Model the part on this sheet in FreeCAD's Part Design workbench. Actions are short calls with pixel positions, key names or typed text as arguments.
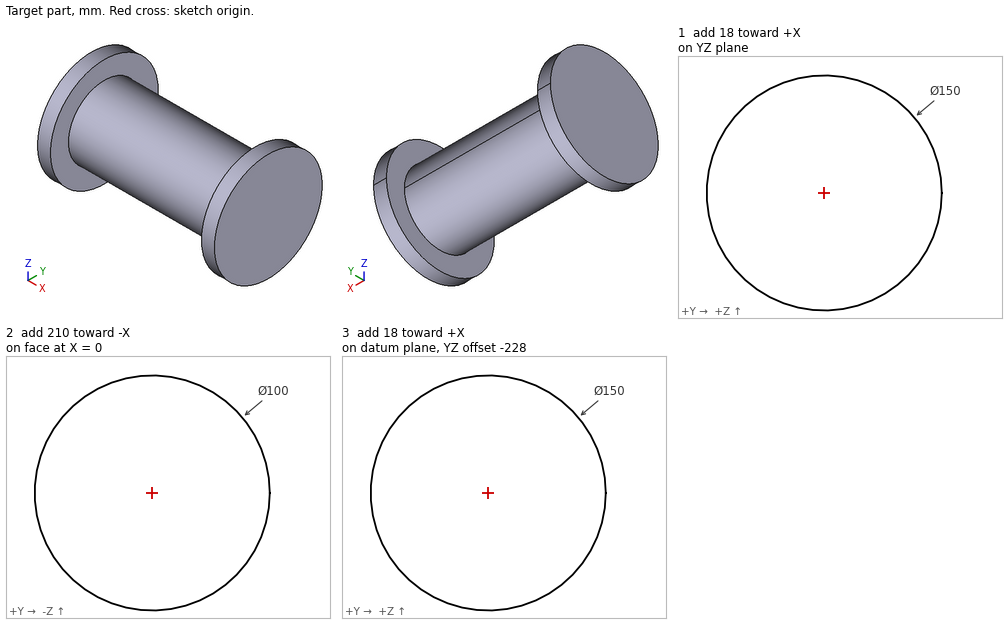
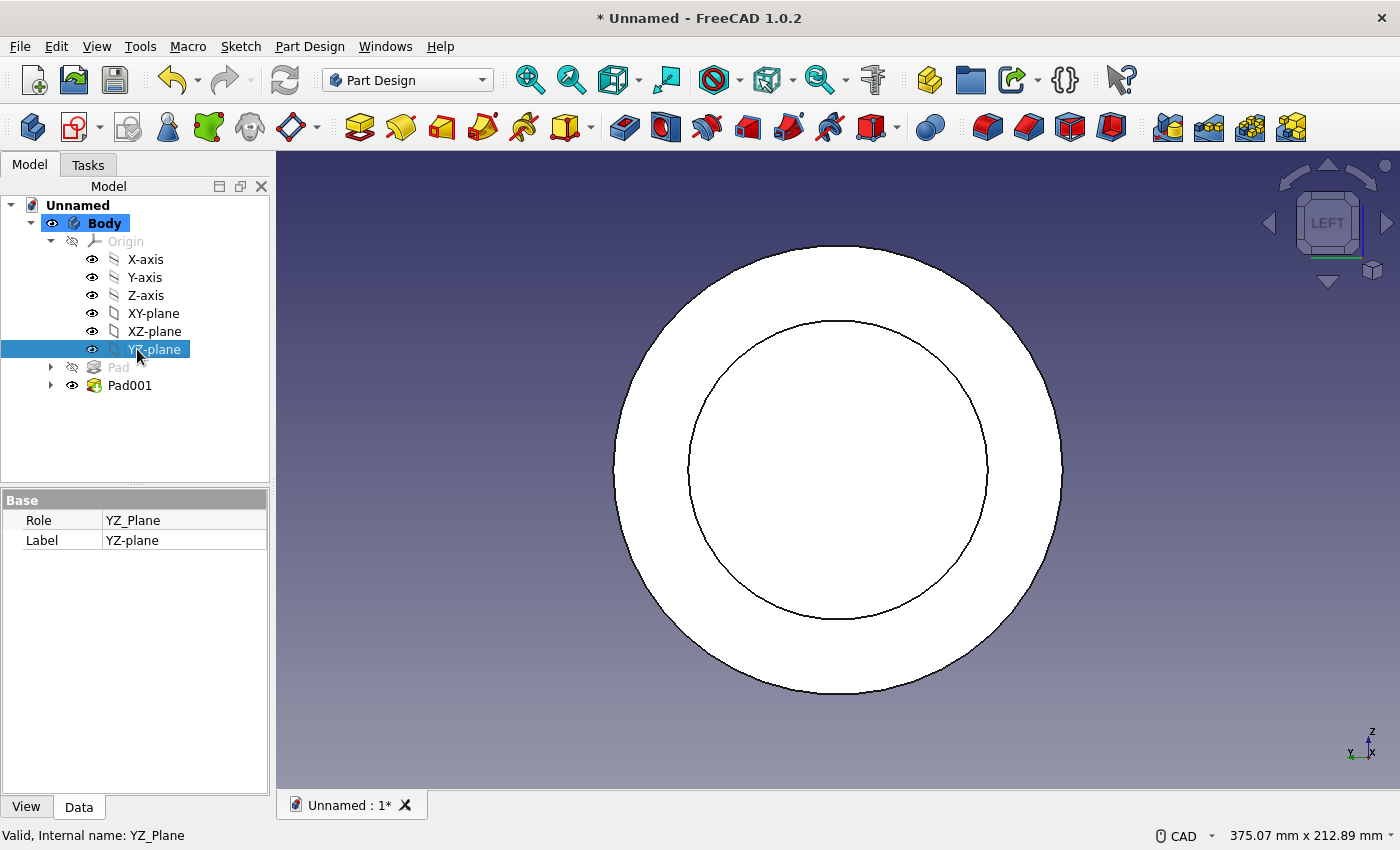
click(290, 128)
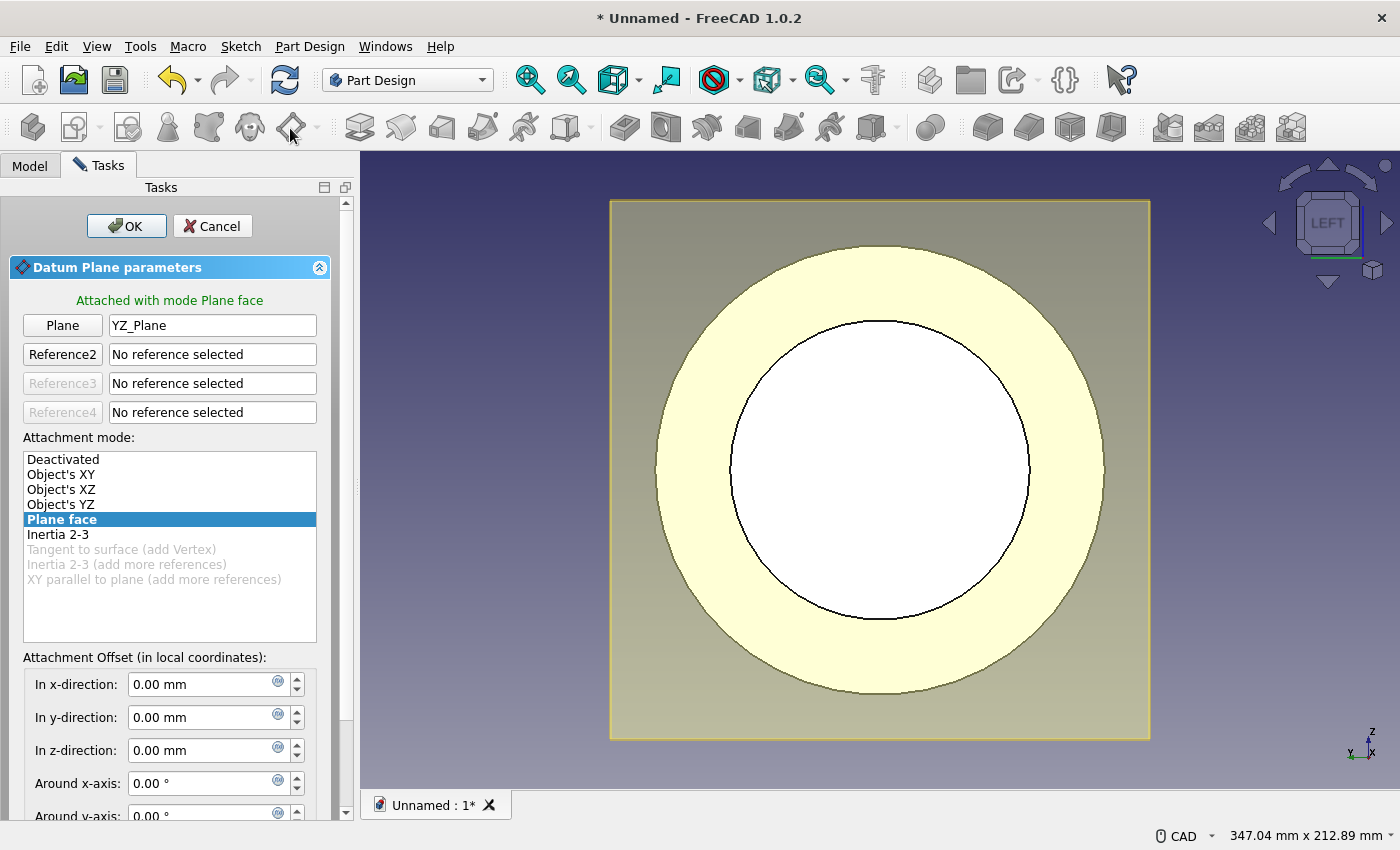
triple_click(210, 750)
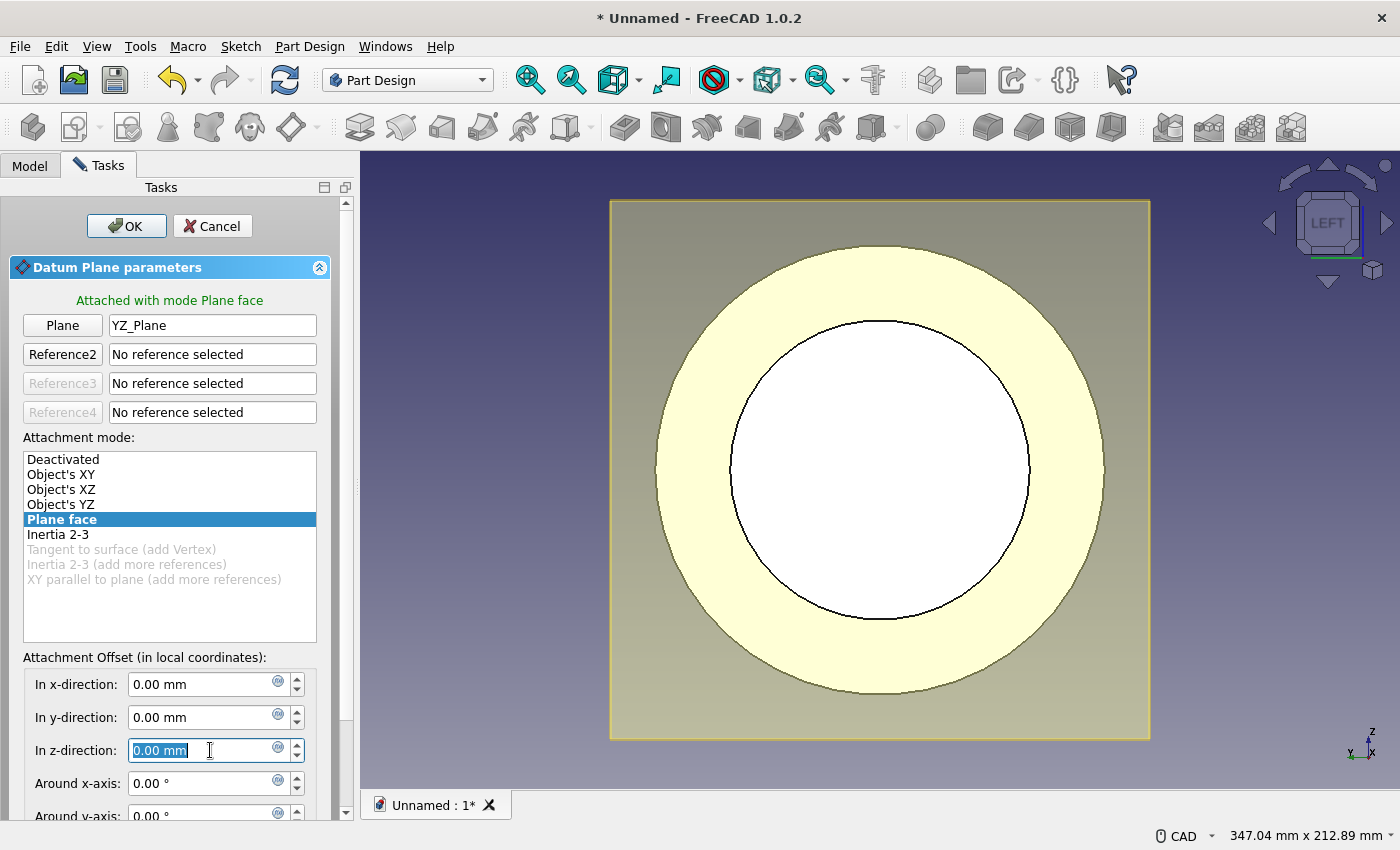
text(-228)
key(Tab)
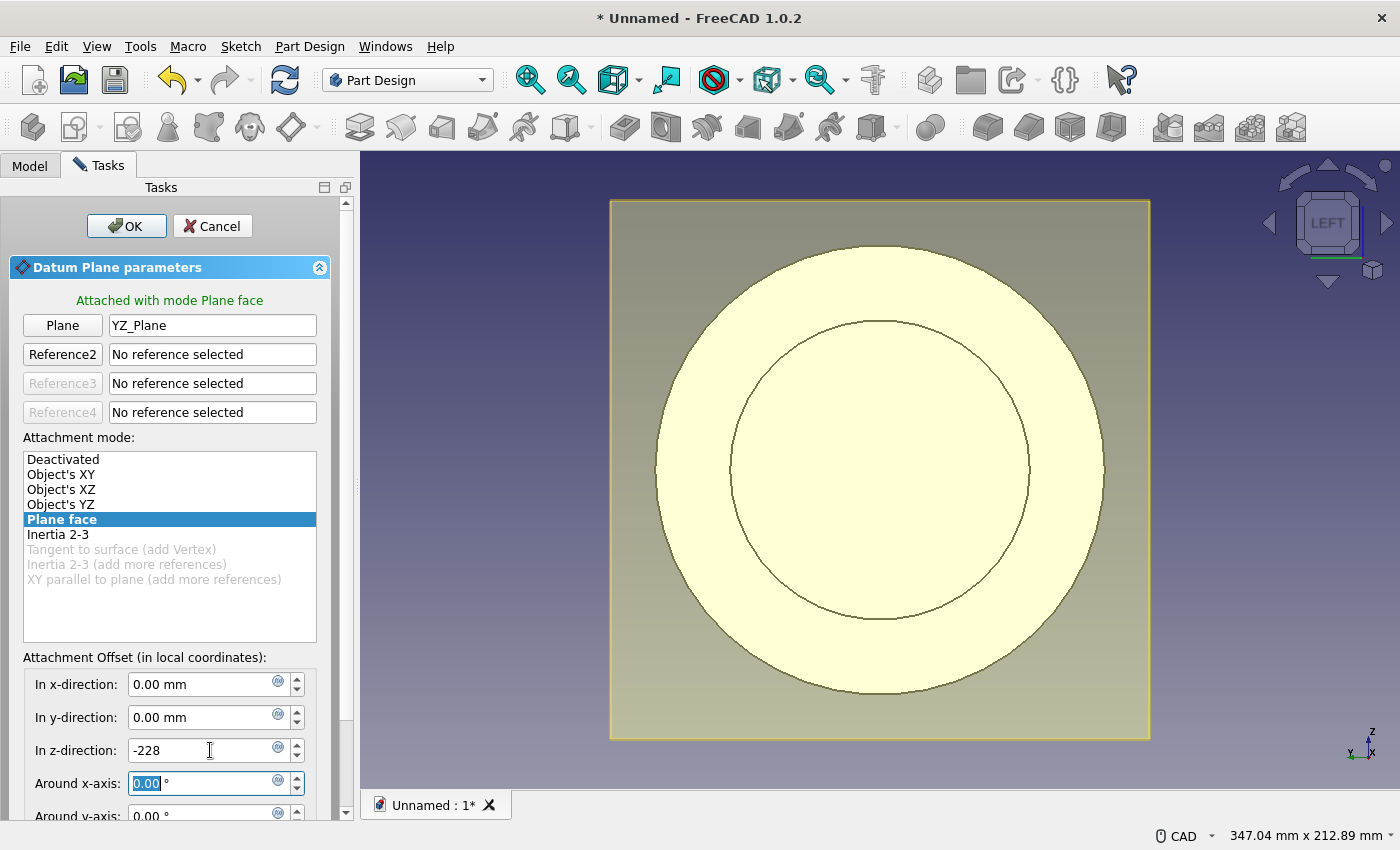
click(127, 226)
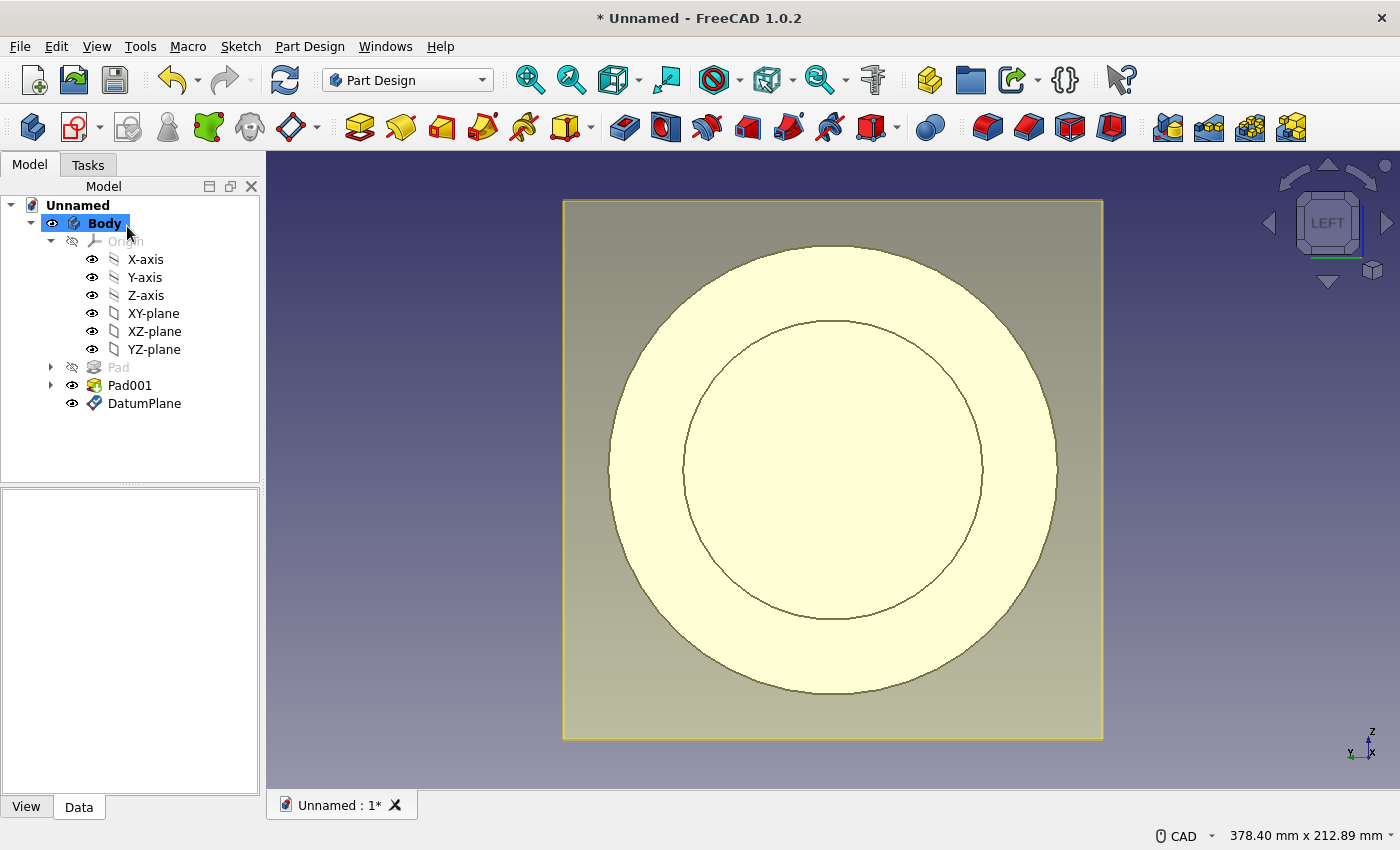
click(117, 403)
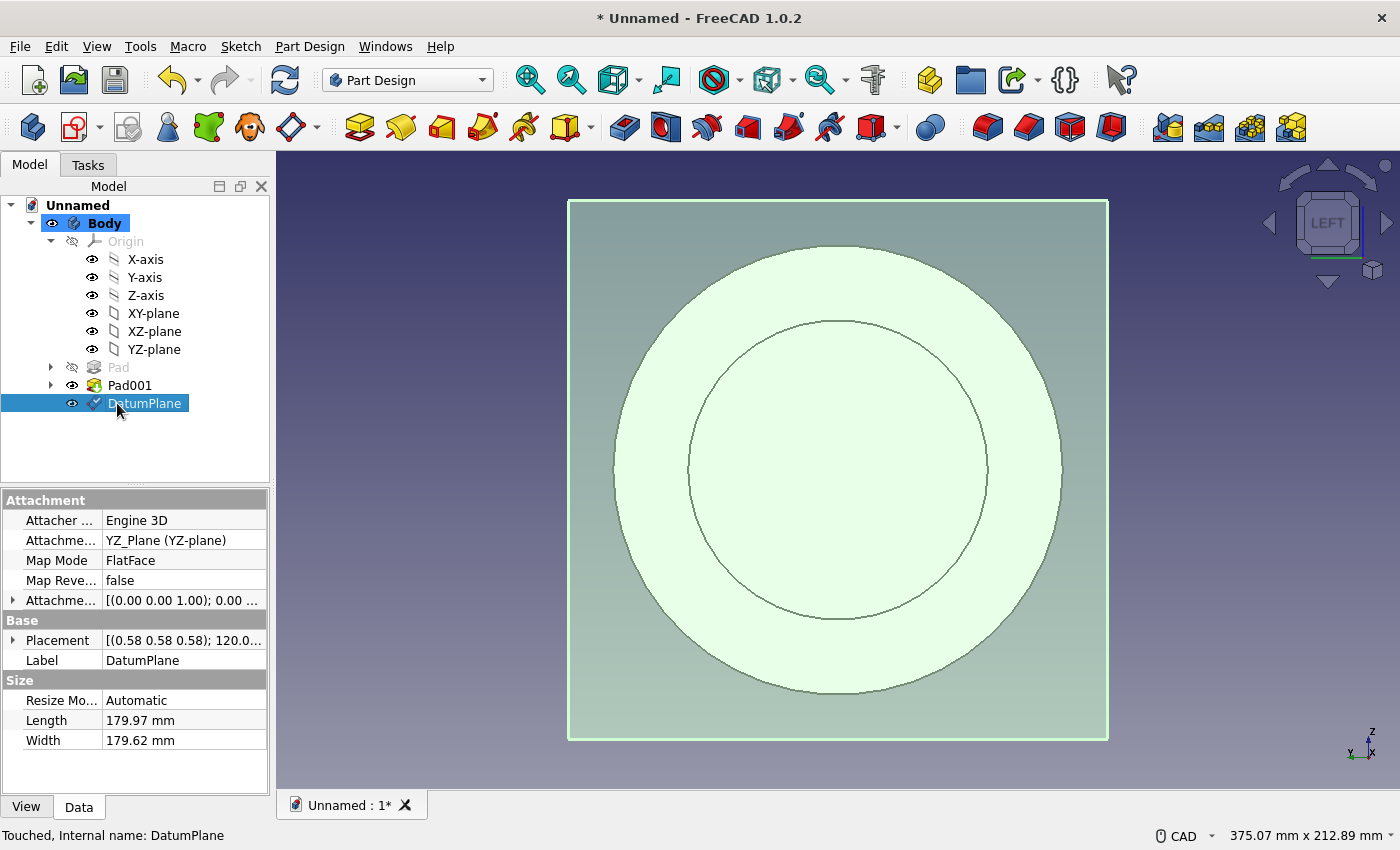
click(74, 128)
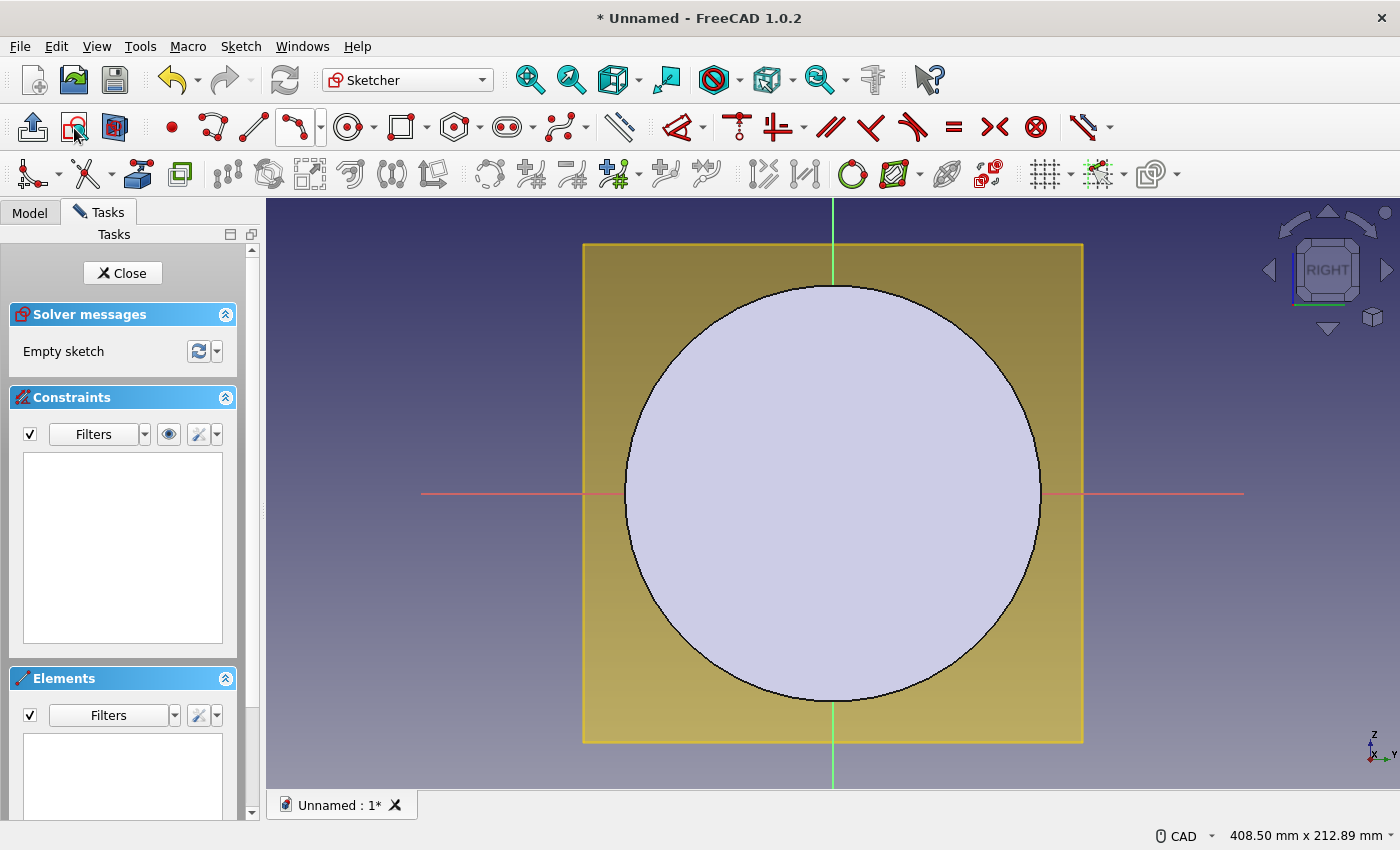
key(q)
key(s)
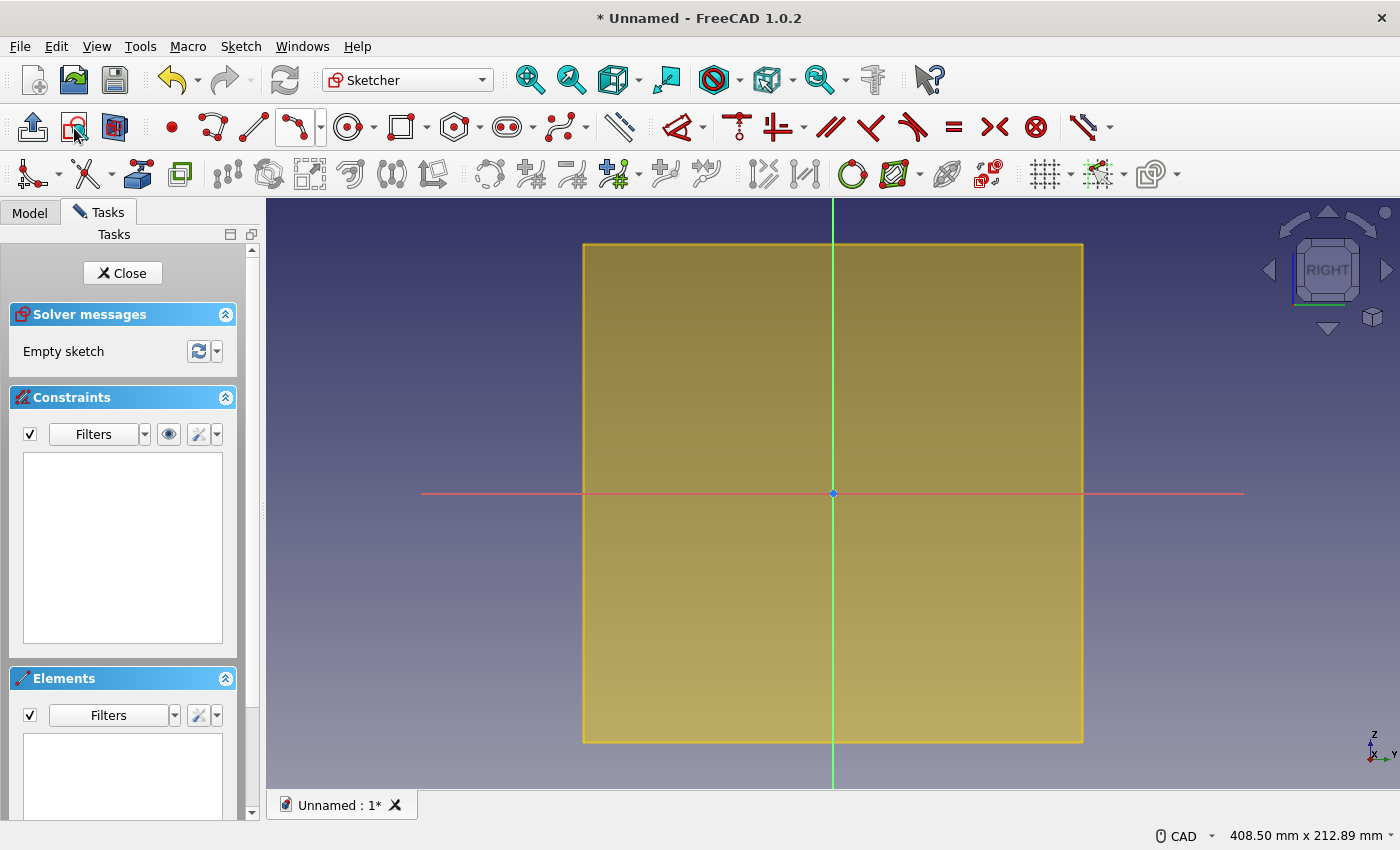
click(348, 128)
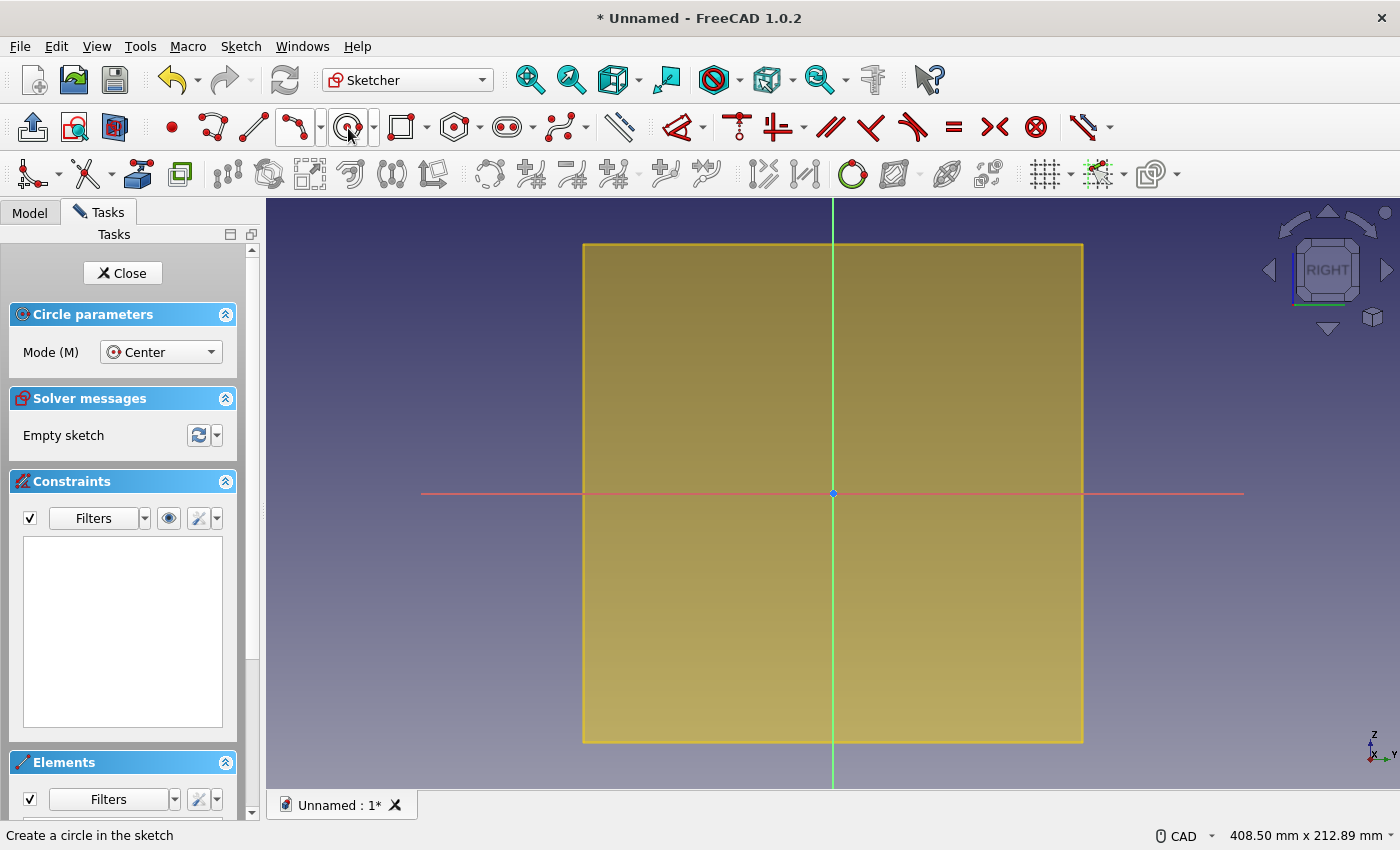
click(833, 494)
move(980, 346)